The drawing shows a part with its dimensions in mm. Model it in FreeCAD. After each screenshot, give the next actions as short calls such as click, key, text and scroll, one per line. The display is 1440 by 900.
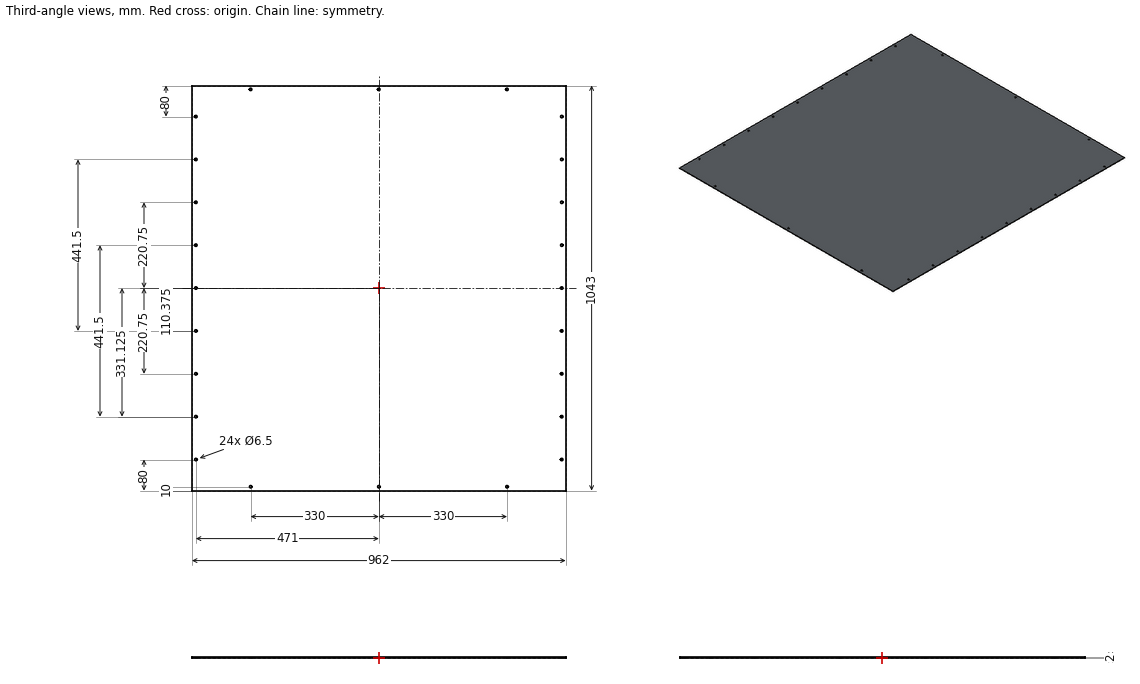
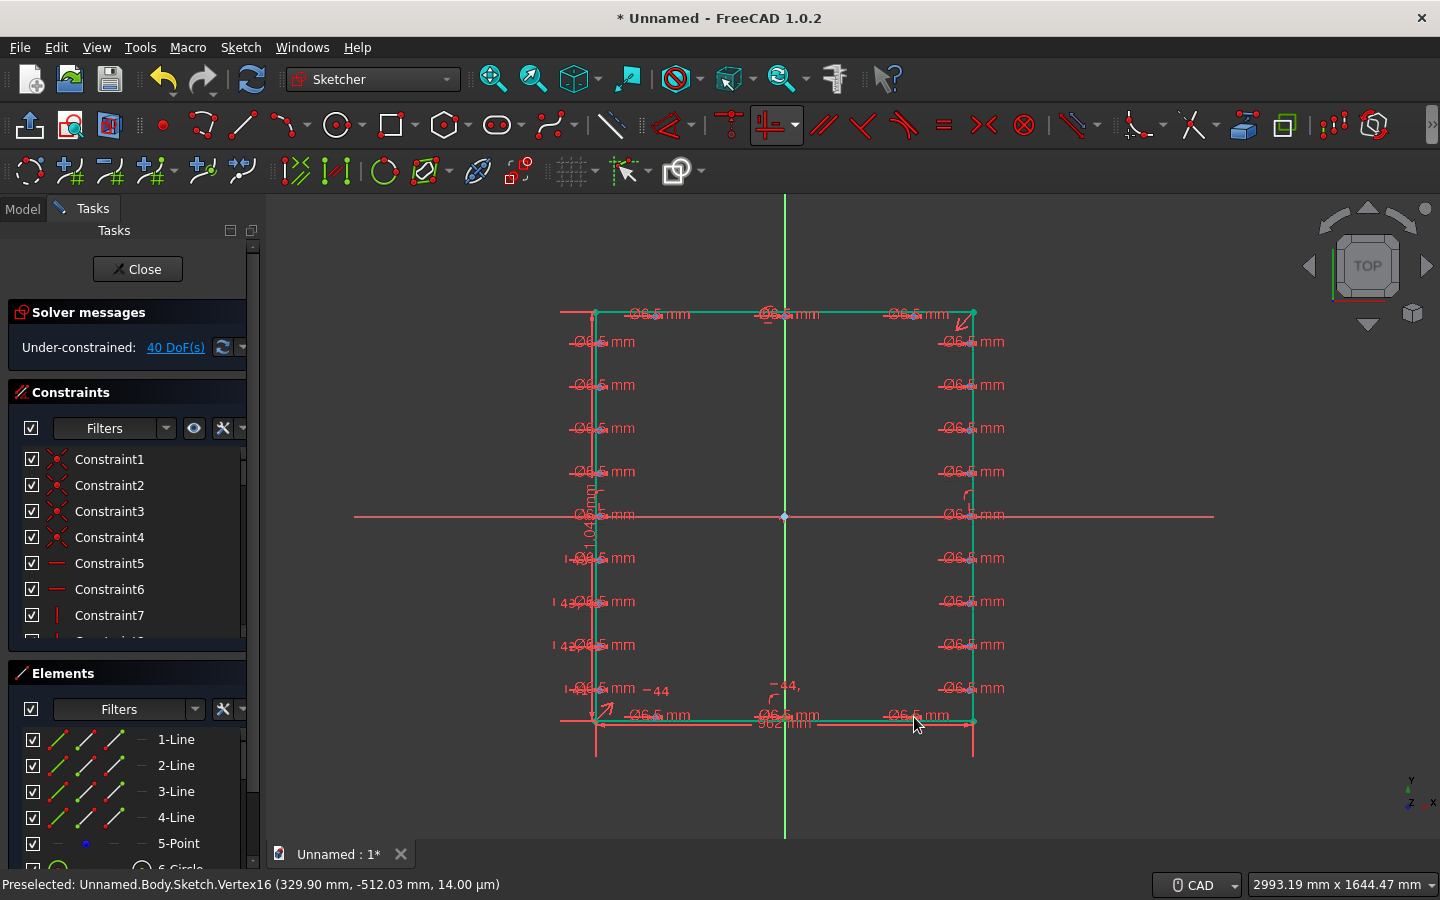
key(h)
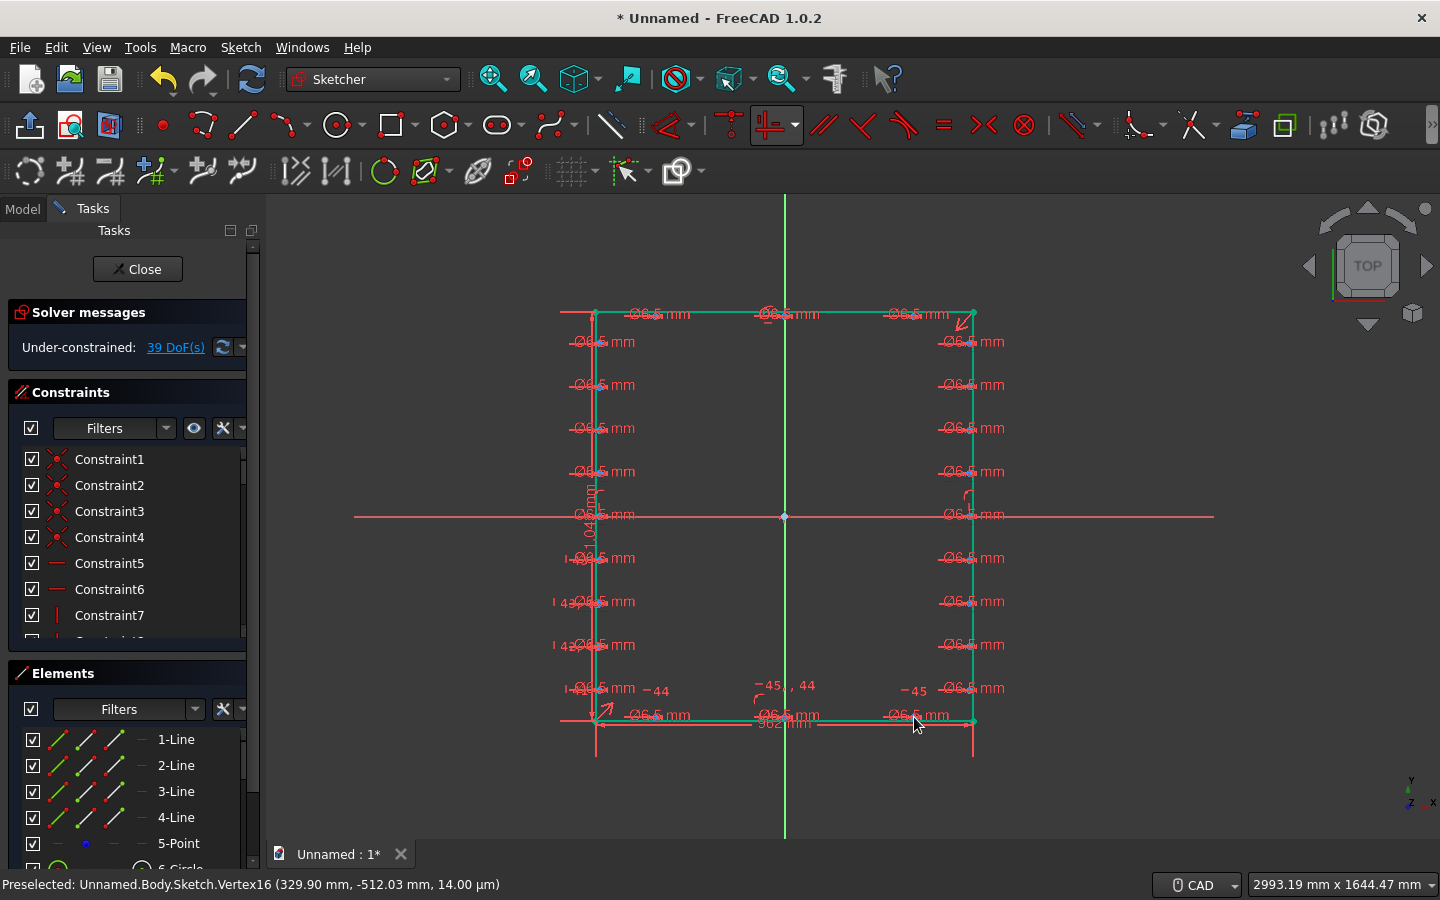
click(600, 690)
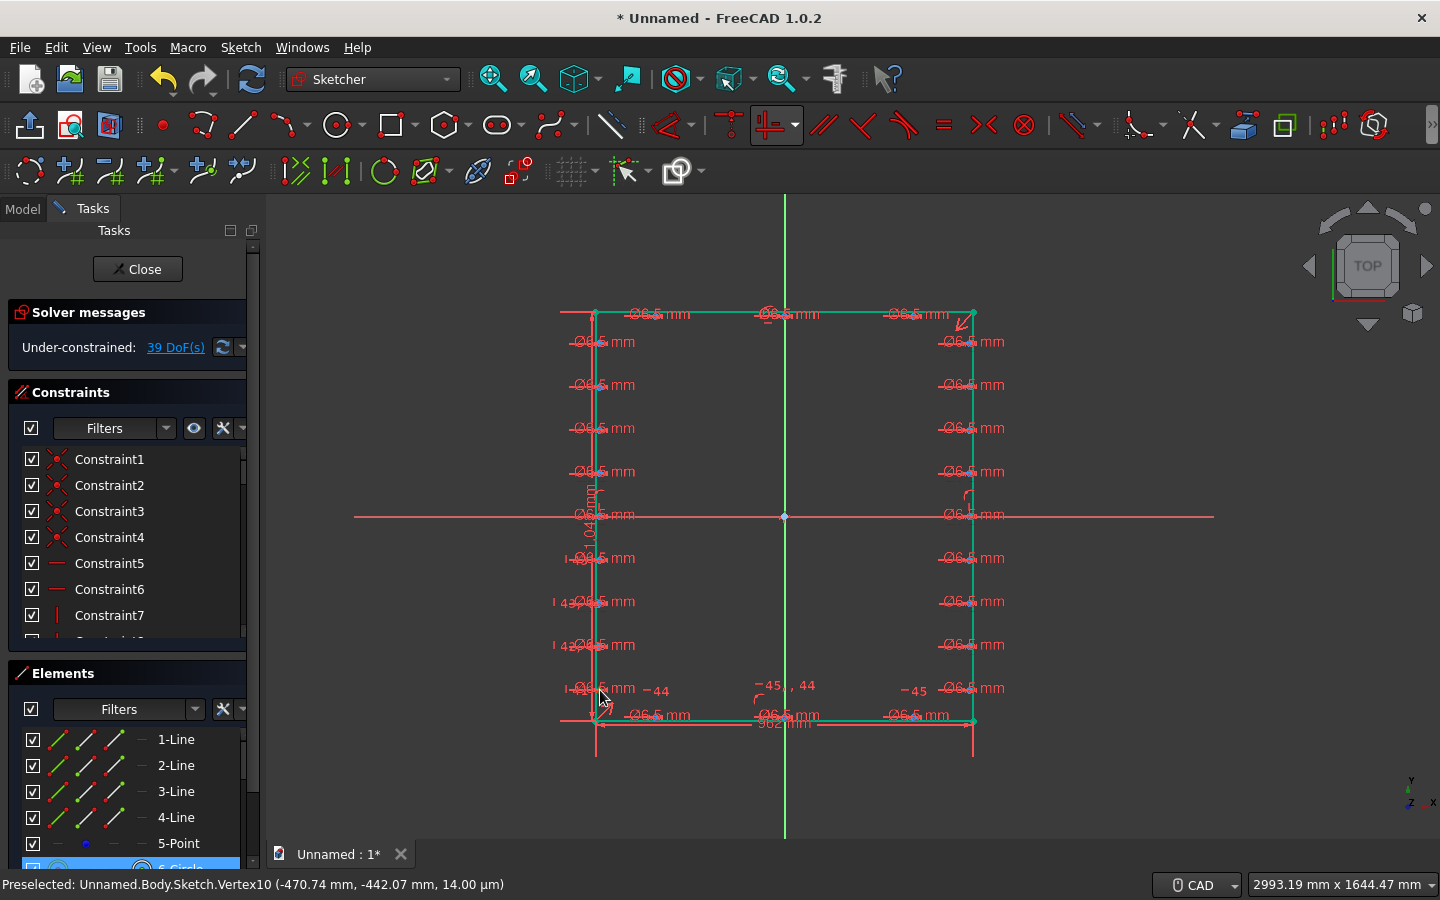
click(969, 690)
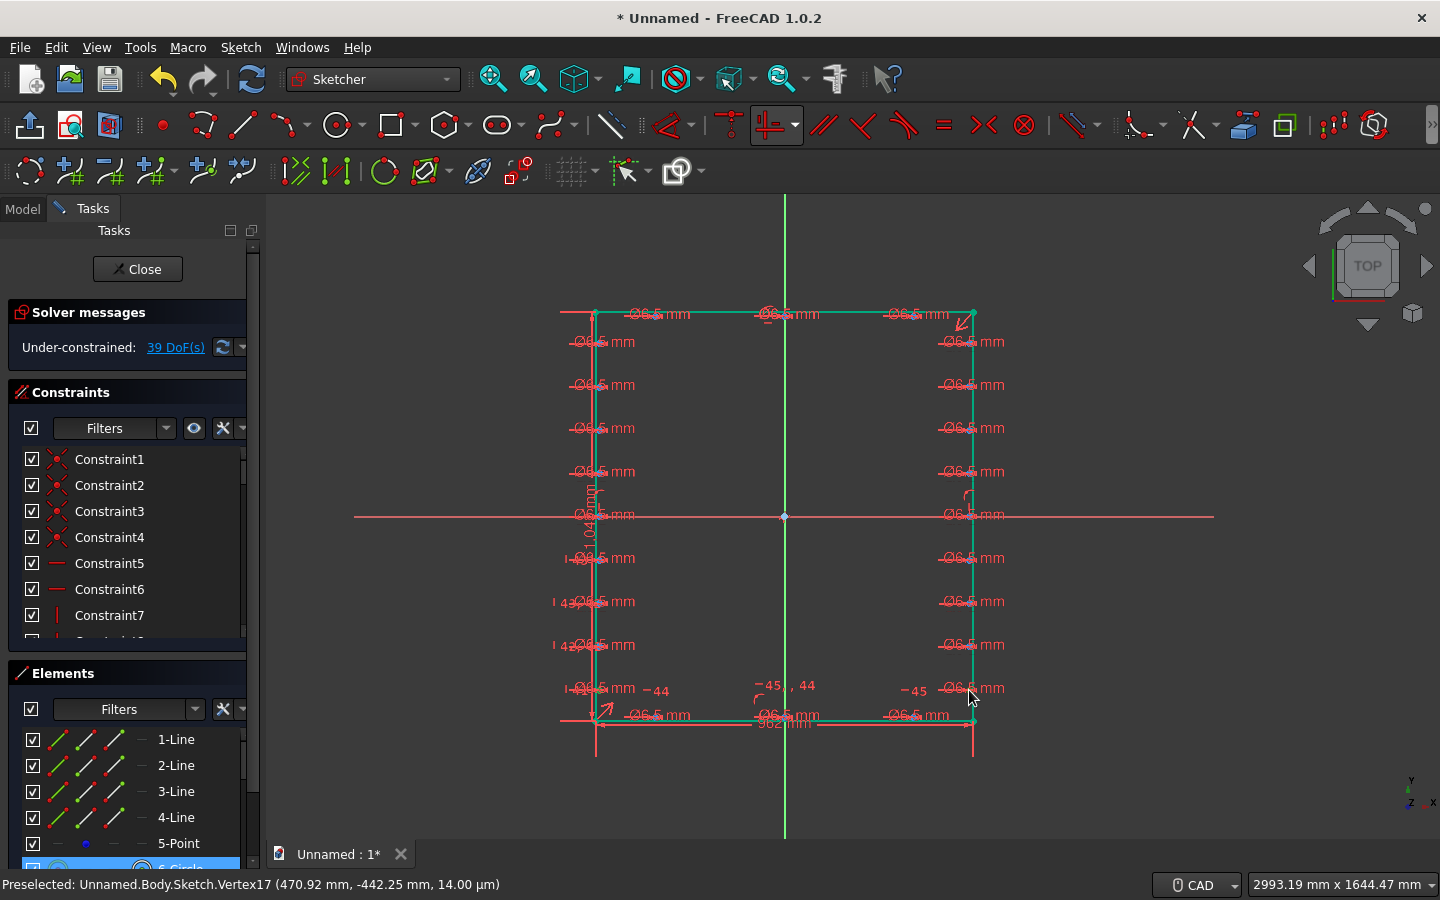
key(h)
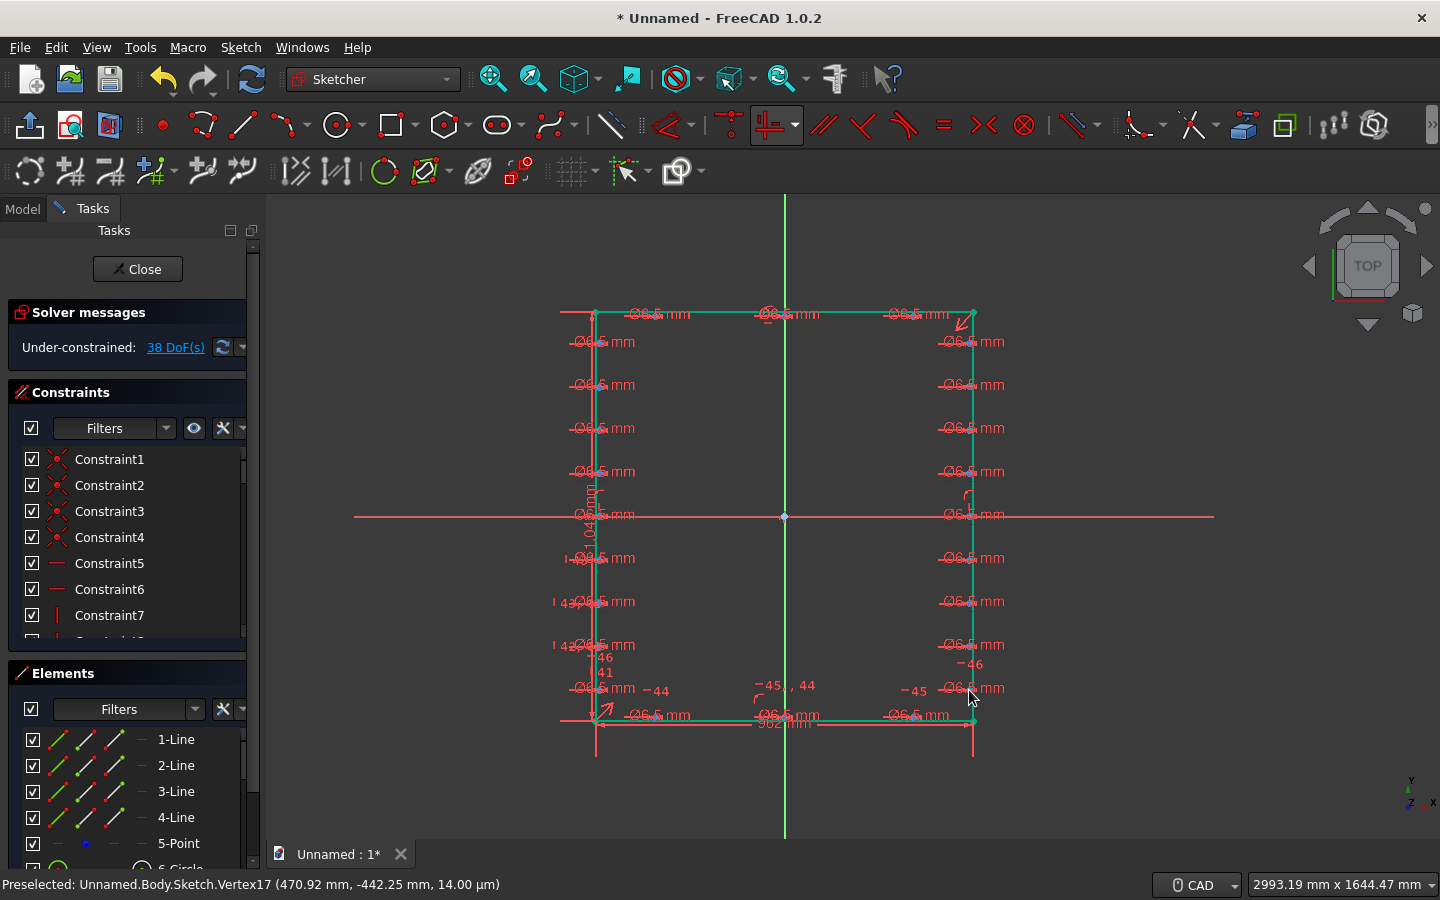
click(969, 690)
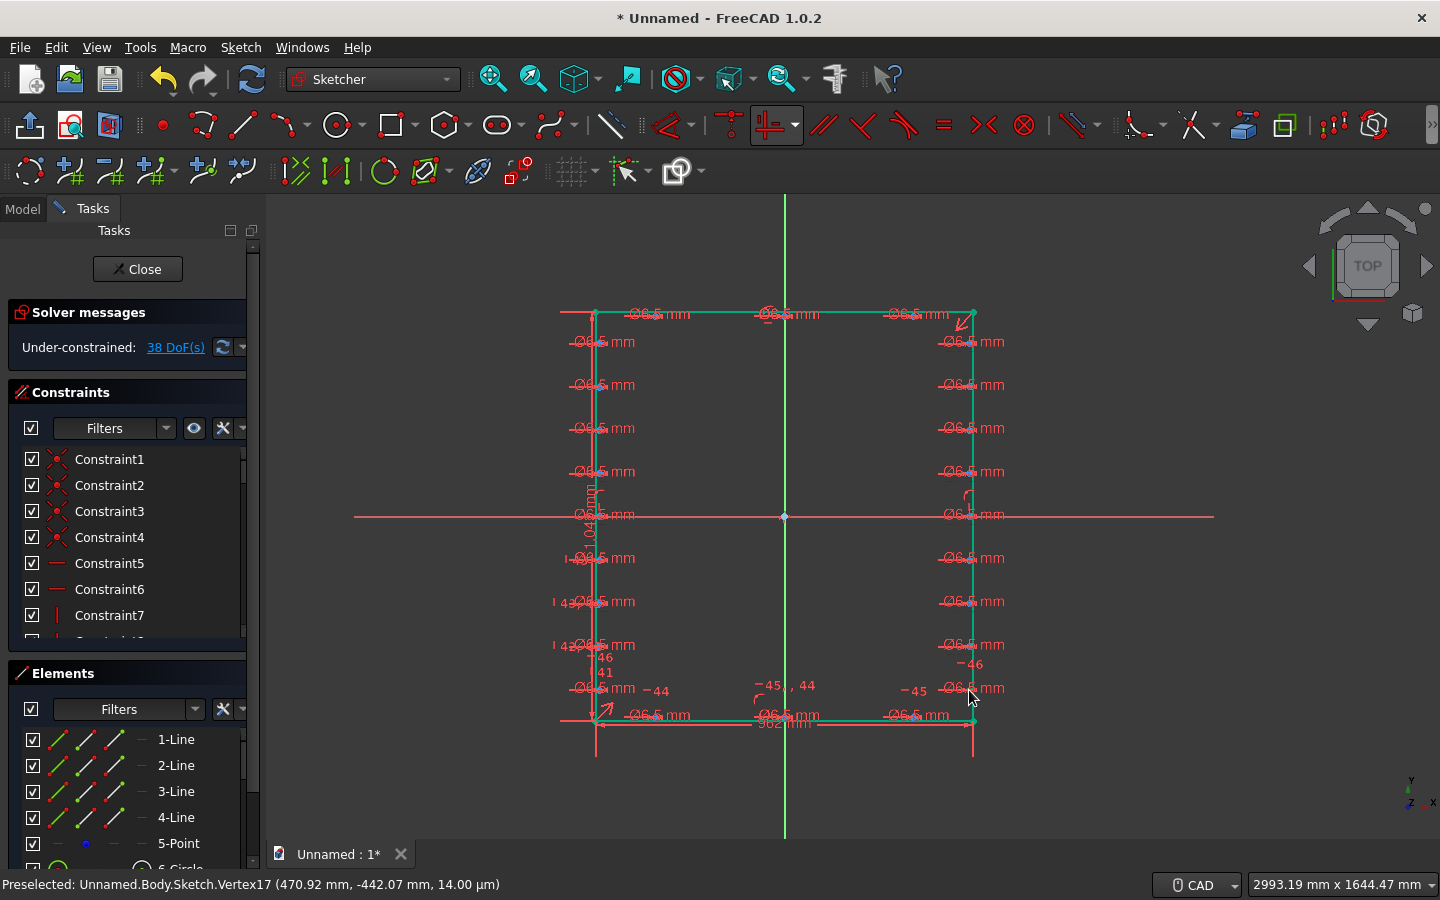
click(969, 647)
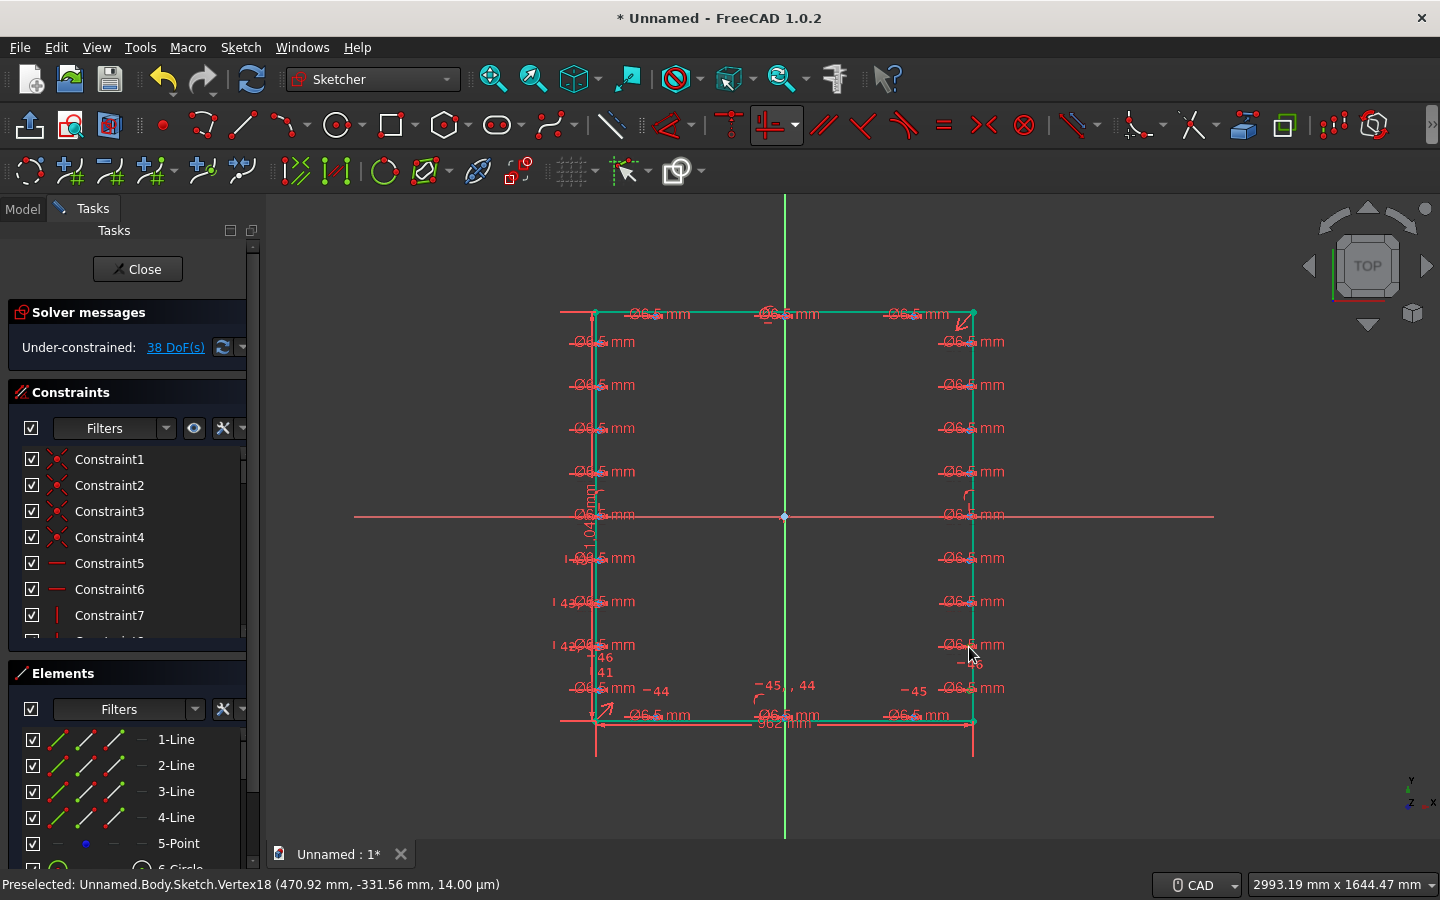
key(v)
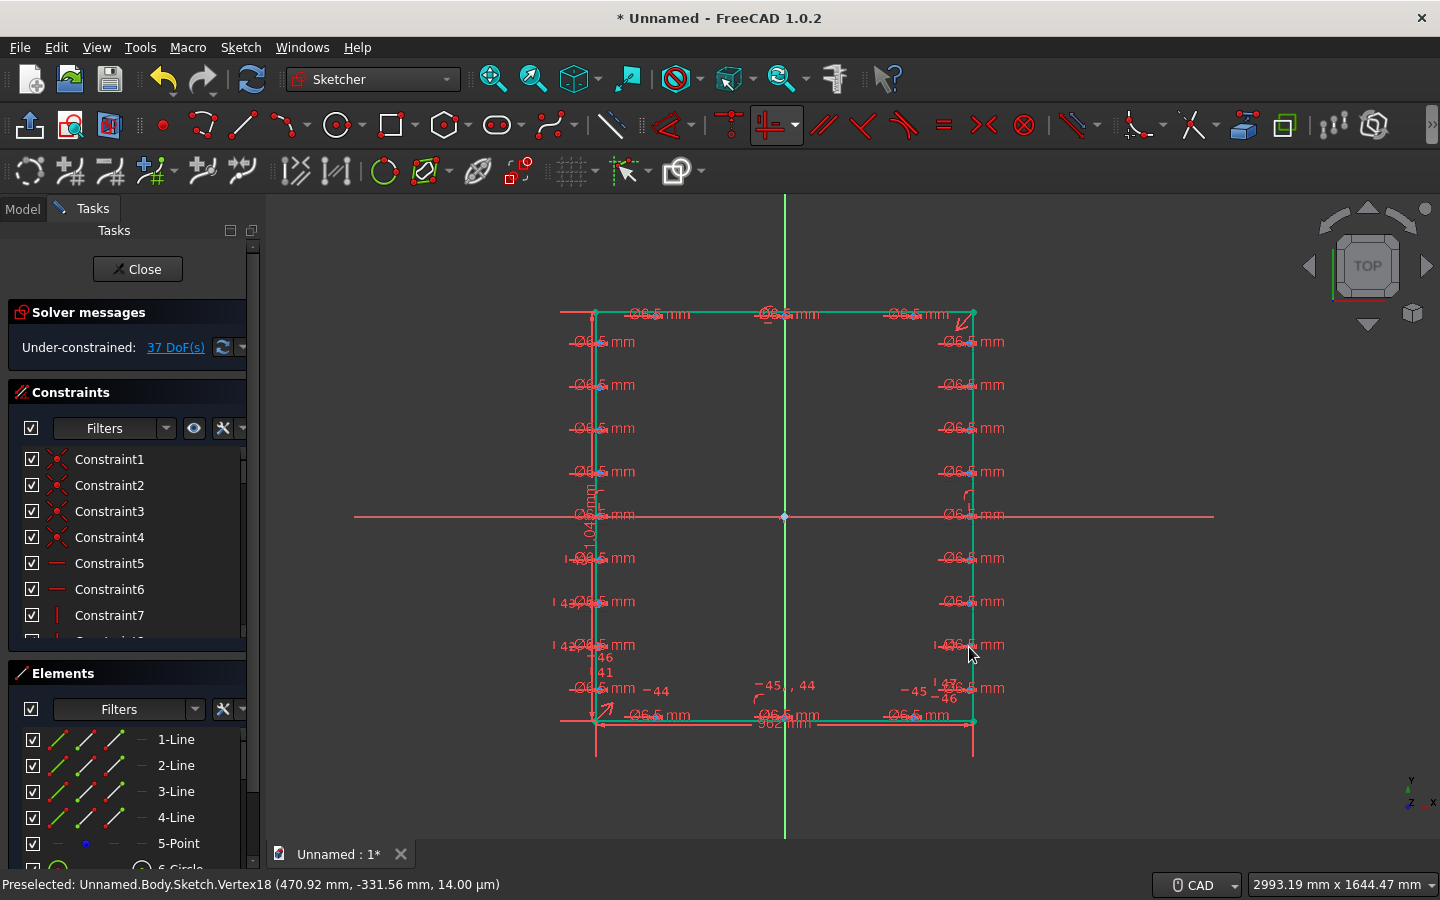
click(969, 647)